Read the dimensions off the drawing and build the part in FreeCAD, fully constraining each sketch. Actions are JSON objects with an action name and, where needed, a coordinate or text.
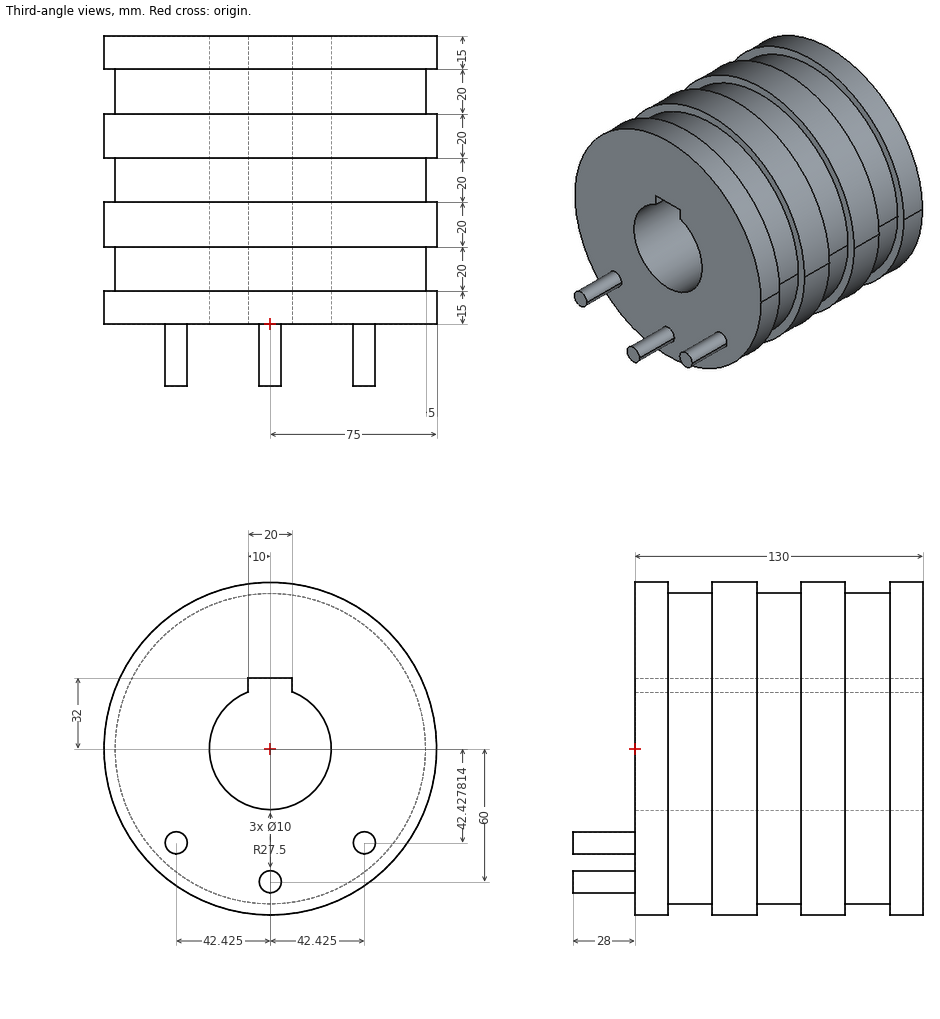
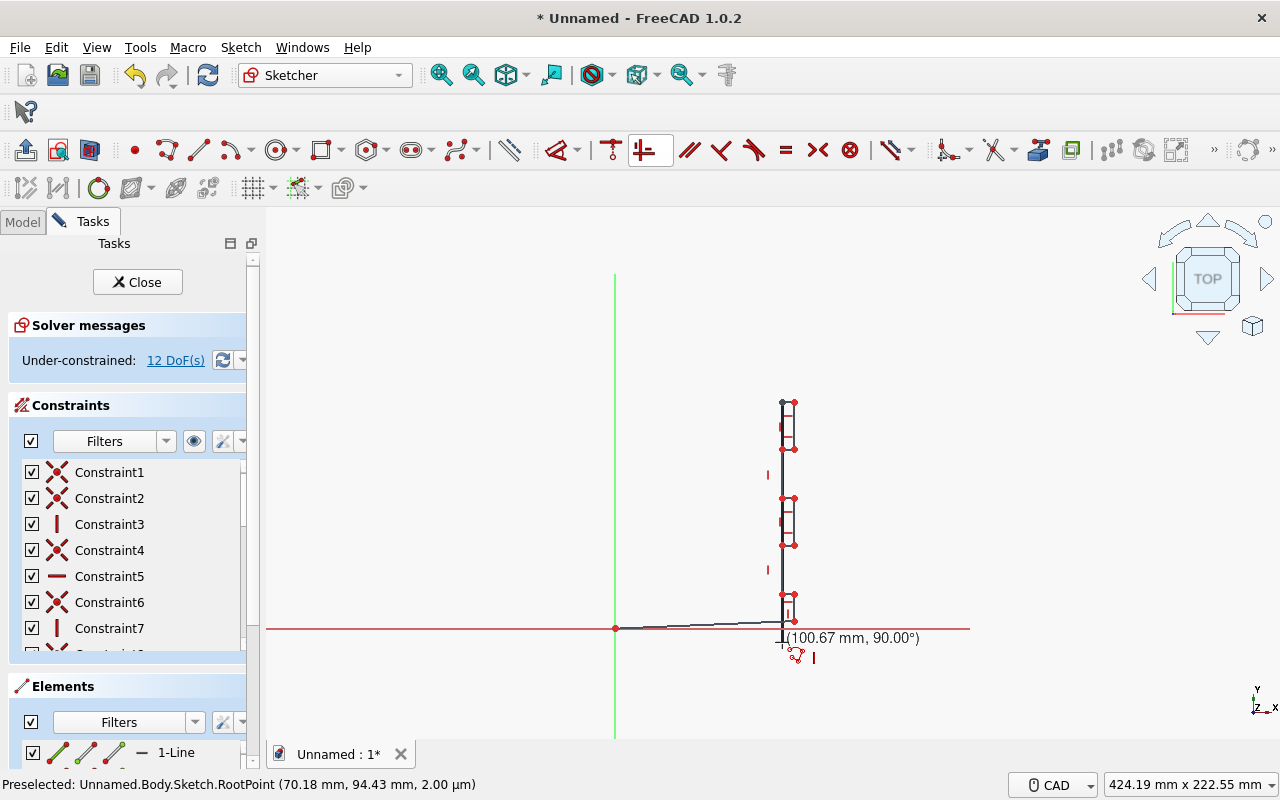
{"action": "left_click", "coordinate": [782, 354]}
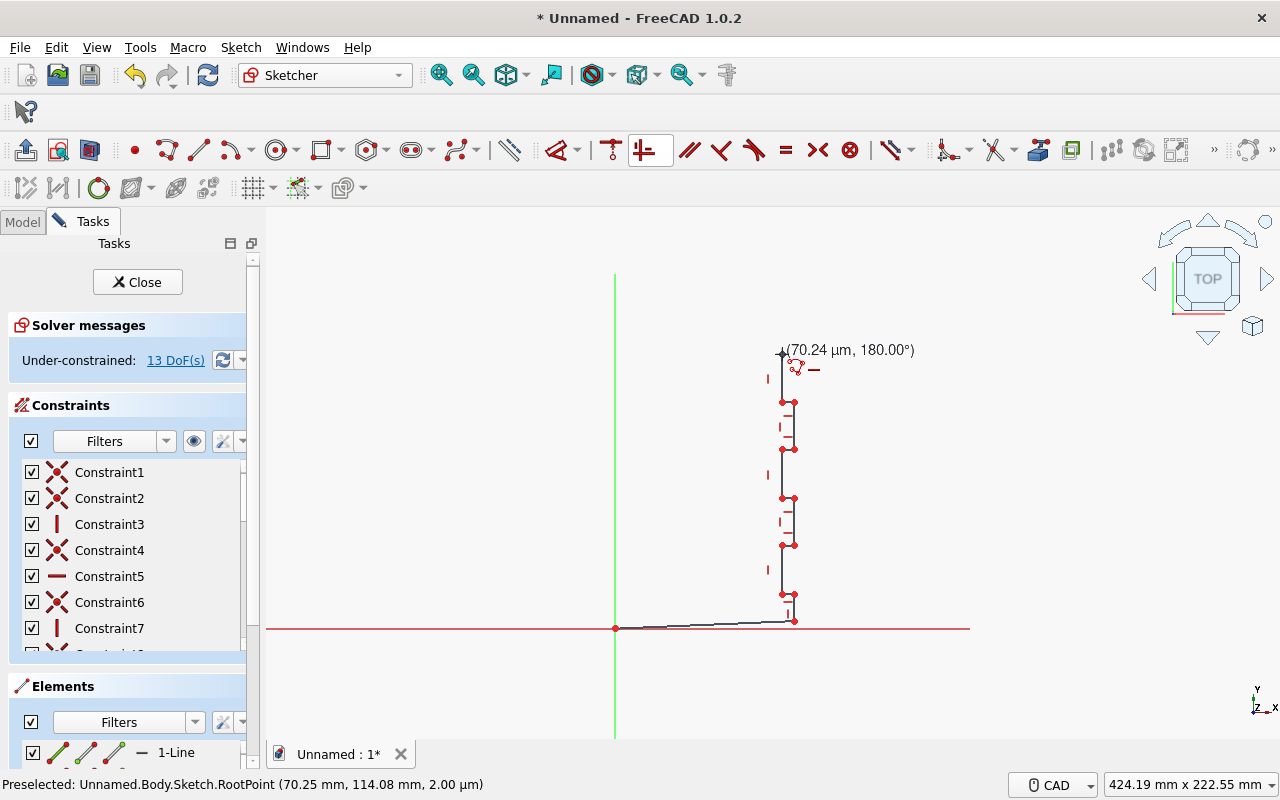
{"action": "scroll", "coordinate": [794, 354], "scroll_direction": "up", "scroll_amount": 2}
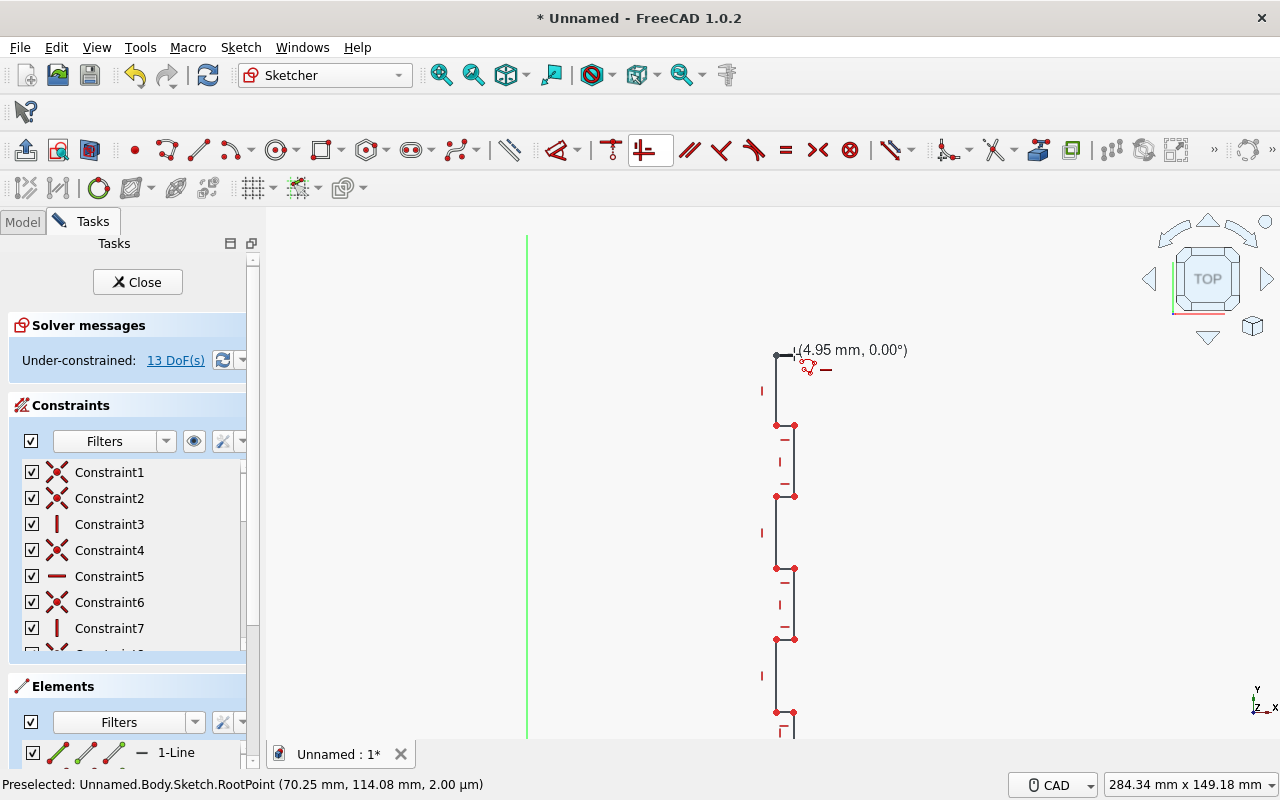
{"action": "left_click", "coordinate": [794, 354]}
{"action": "left_click", "coordinate": [794, 300]}
{"action": "left_click", "coordinate": [536, 300]}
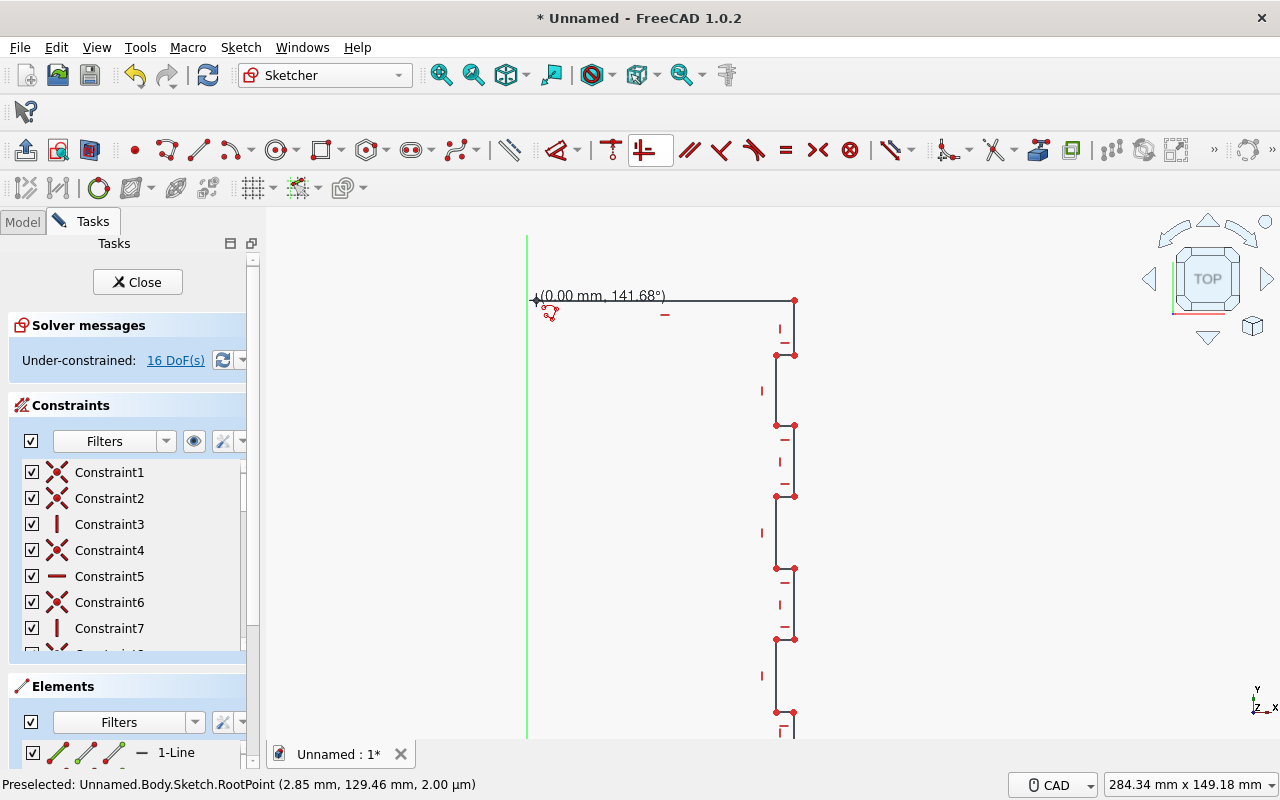
{"action": "scroll", "coordinate": [794, 353], "scroll_direction": "down", "scroll_amount": 2}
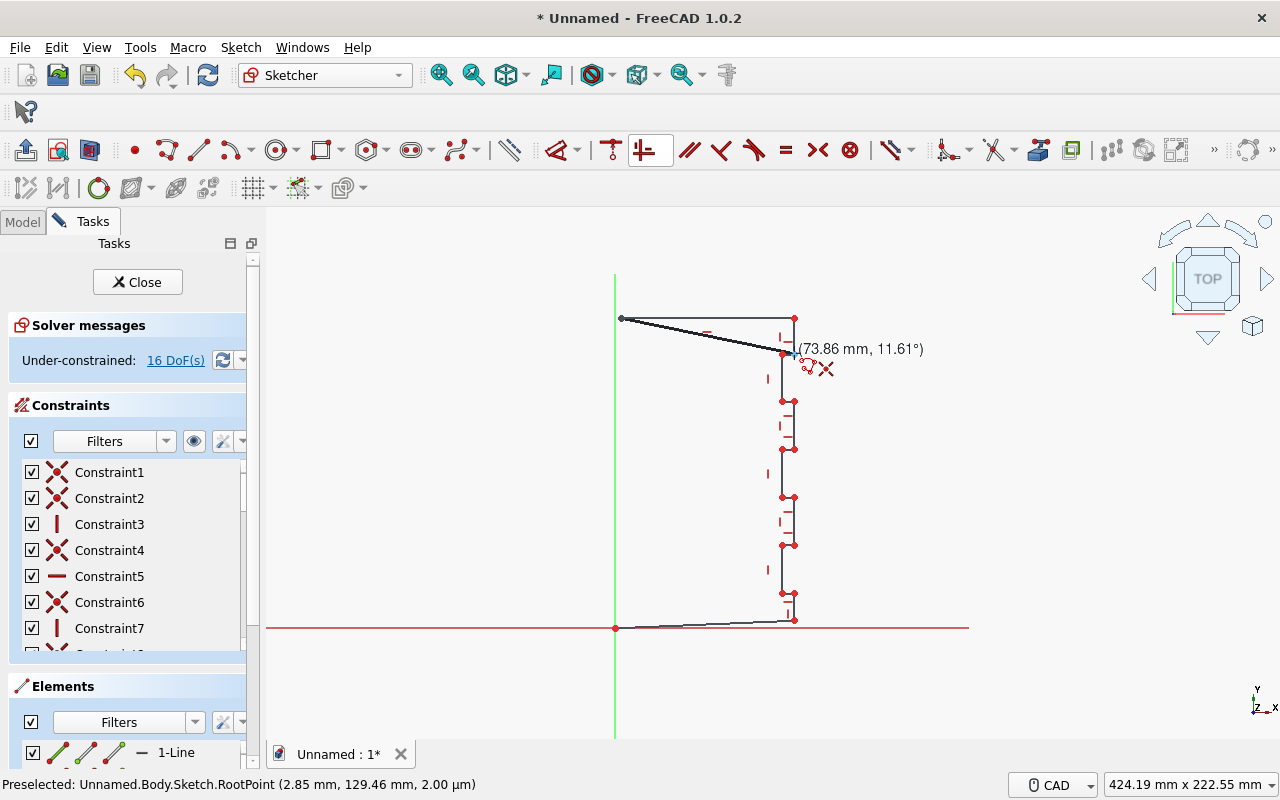
{"action": "left_click", "coordinate": [615, 628]}
{"action": "key", "text": "Escape"}
{"action": "key", "text": "Escape"}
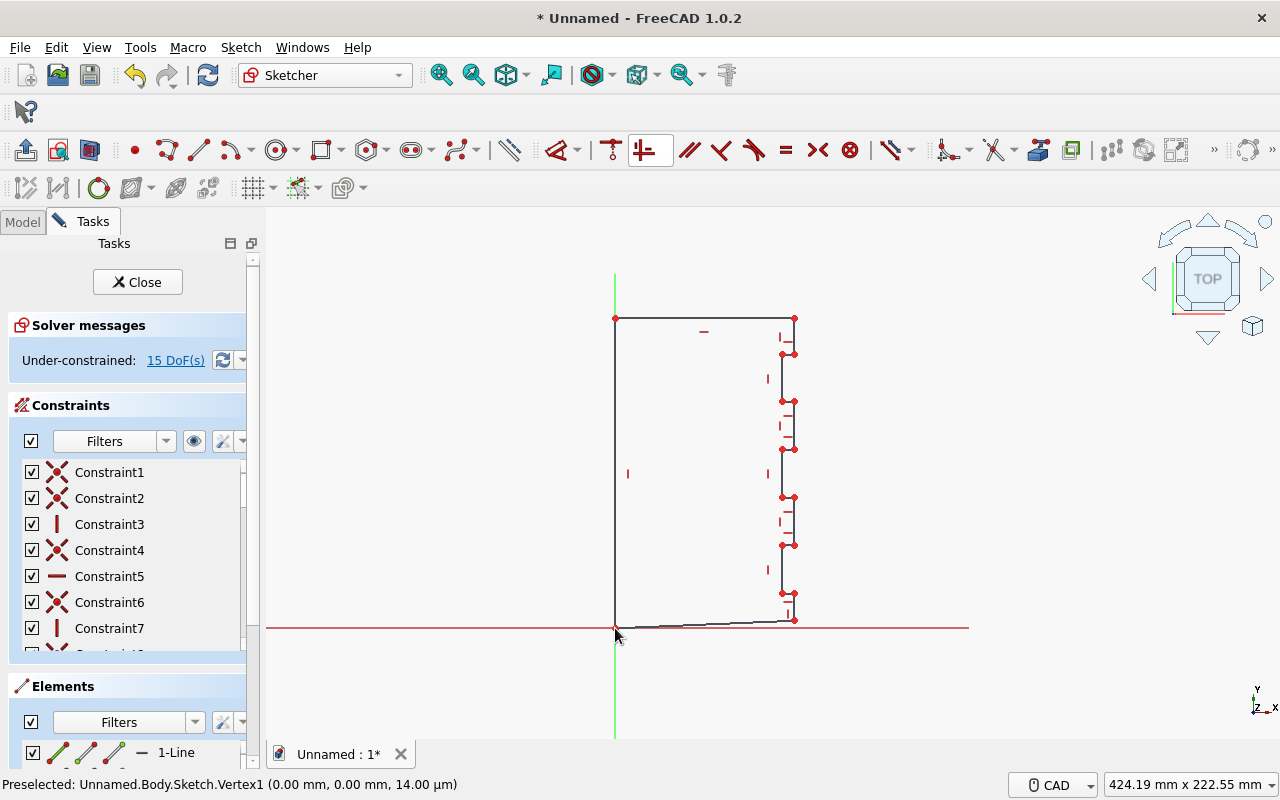
{"action": "left_click", "coordinate": [669, 626]}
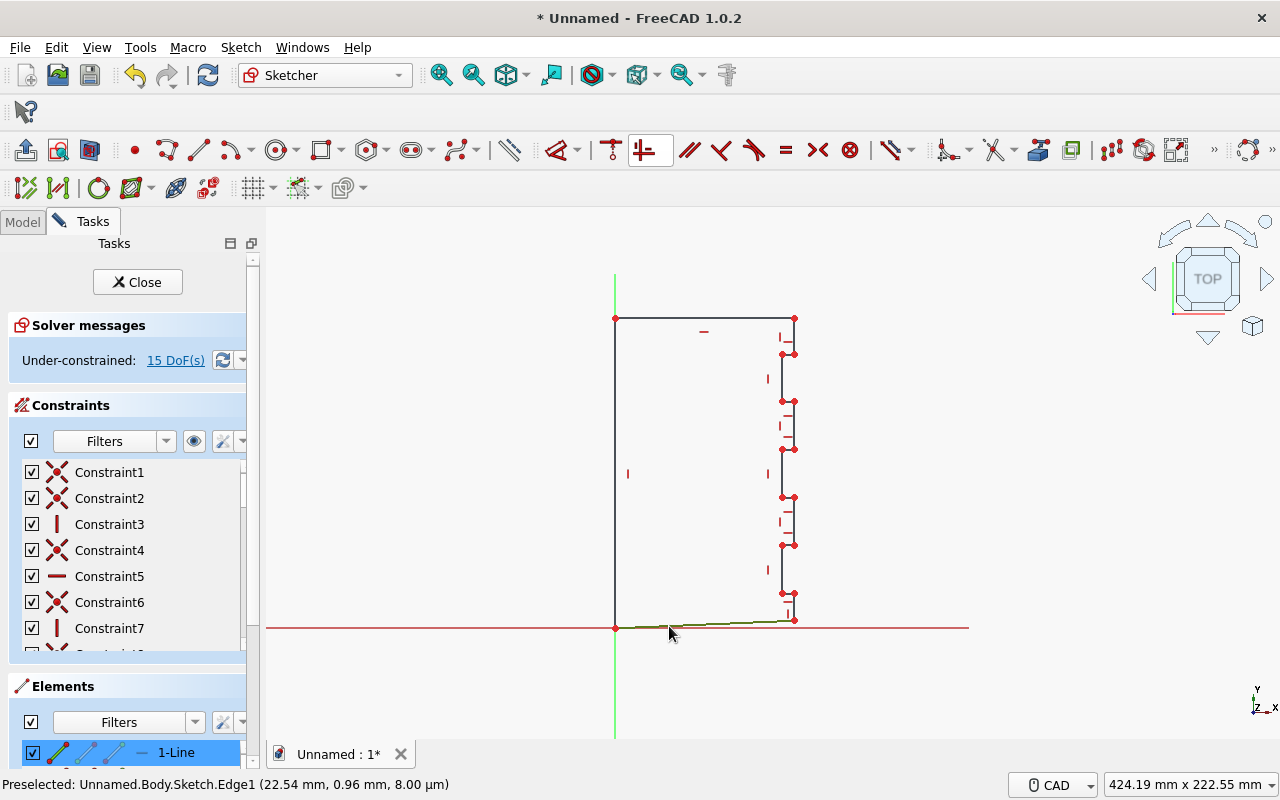
{"action": "key", "text": "h"}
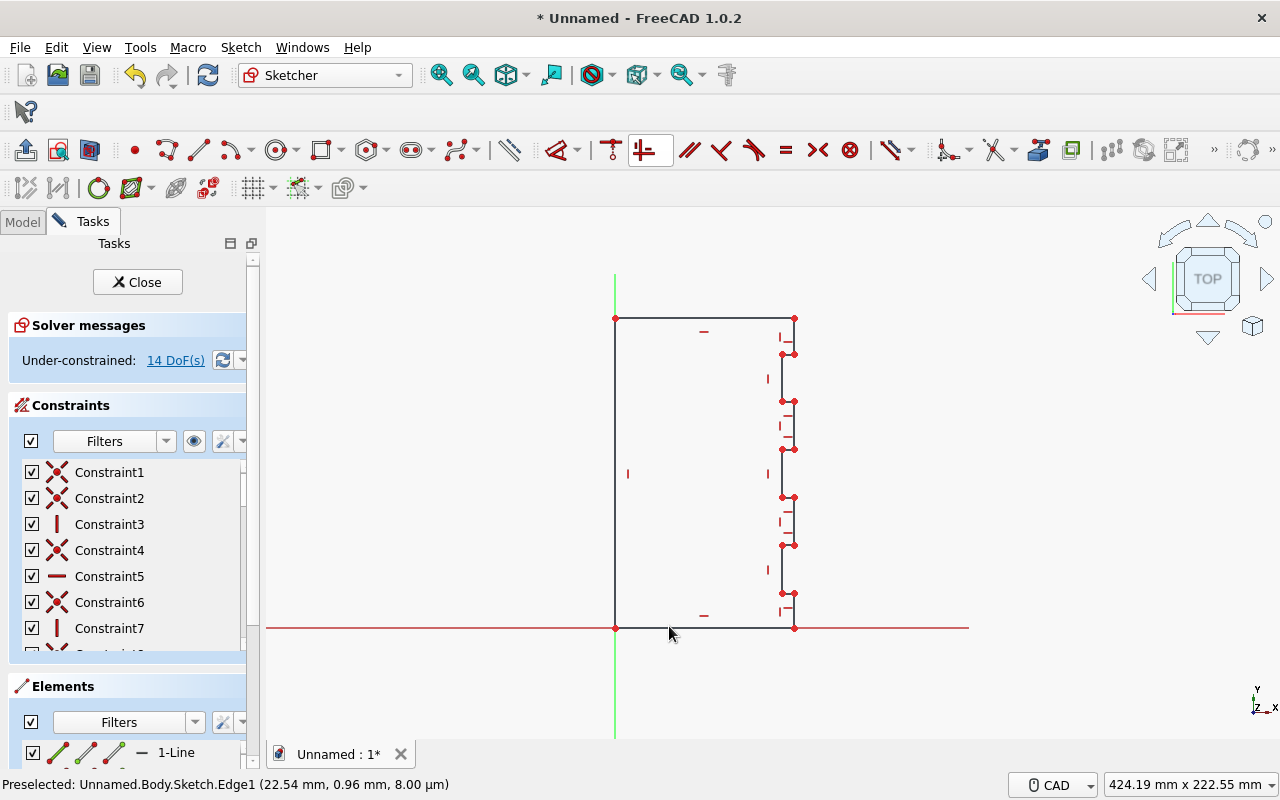
{"action": "scroll", "coordinate": [788, 594], "scroll_direction": "up", "scroll_amount": 7}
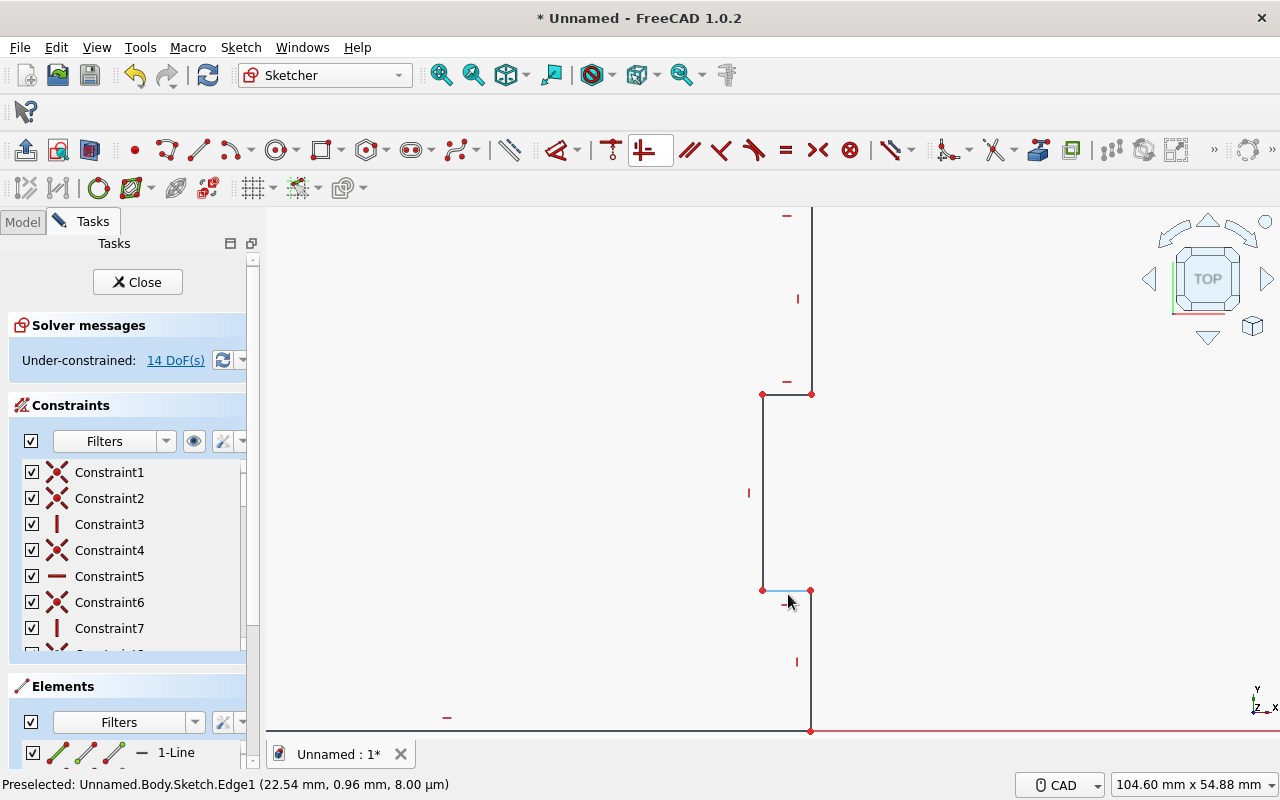
{"action": "left_click", "coordinate": [787, 591]}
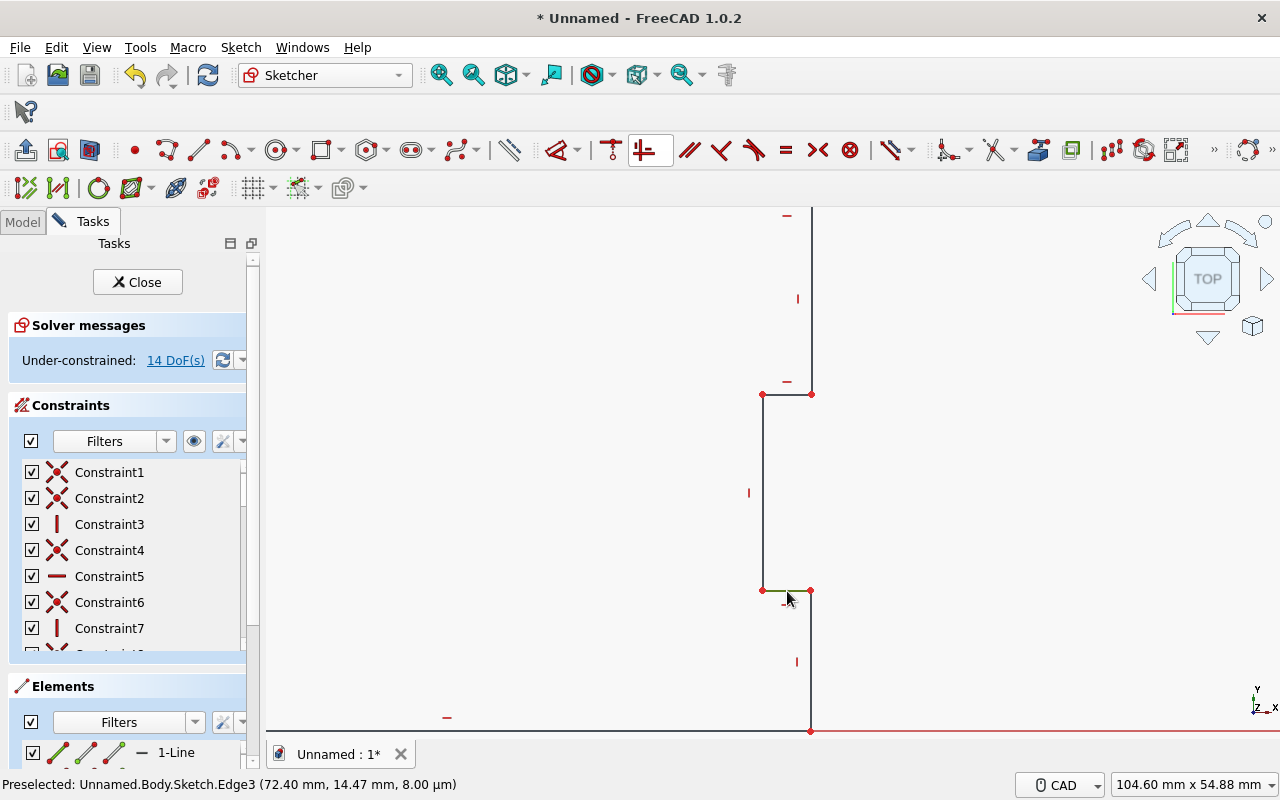
{"action": "key", "text": "l"}